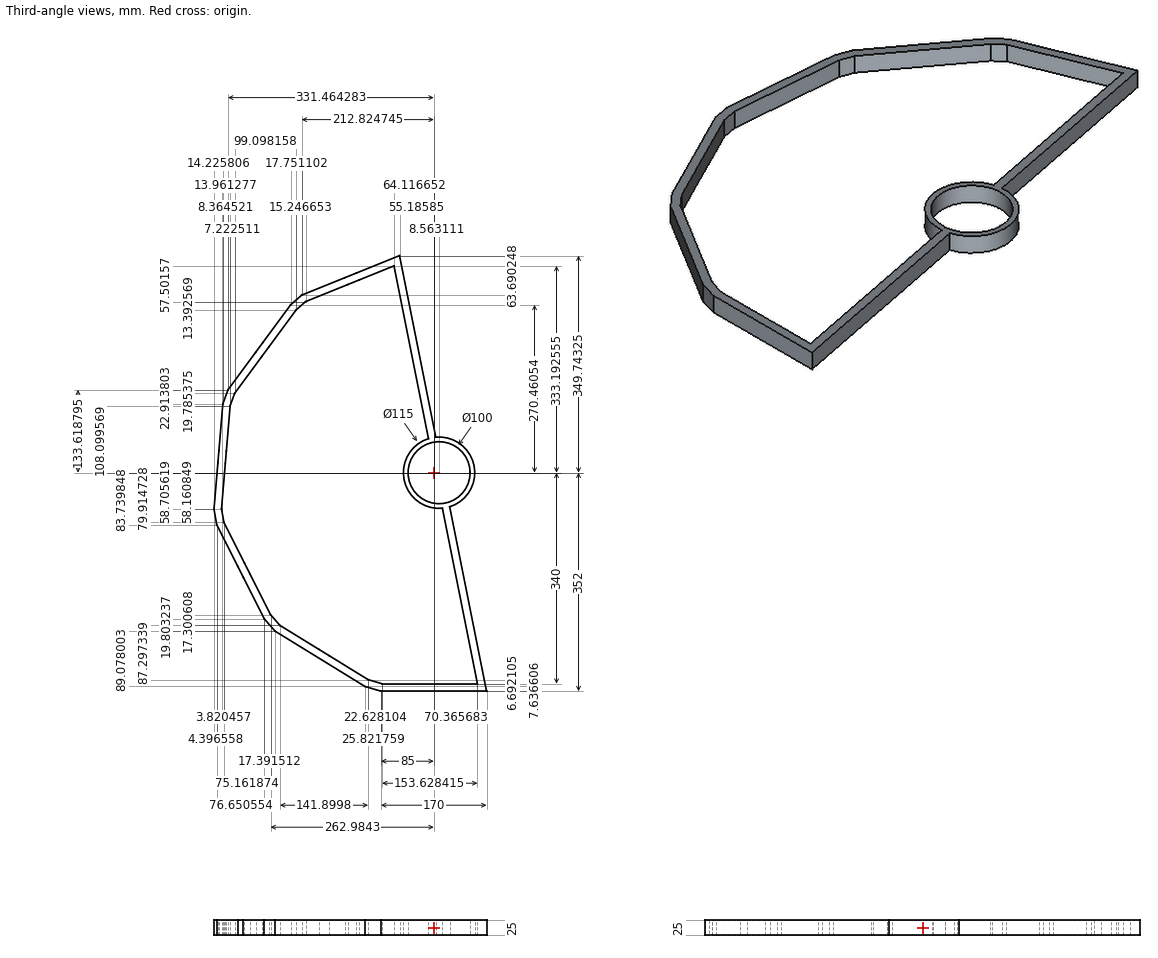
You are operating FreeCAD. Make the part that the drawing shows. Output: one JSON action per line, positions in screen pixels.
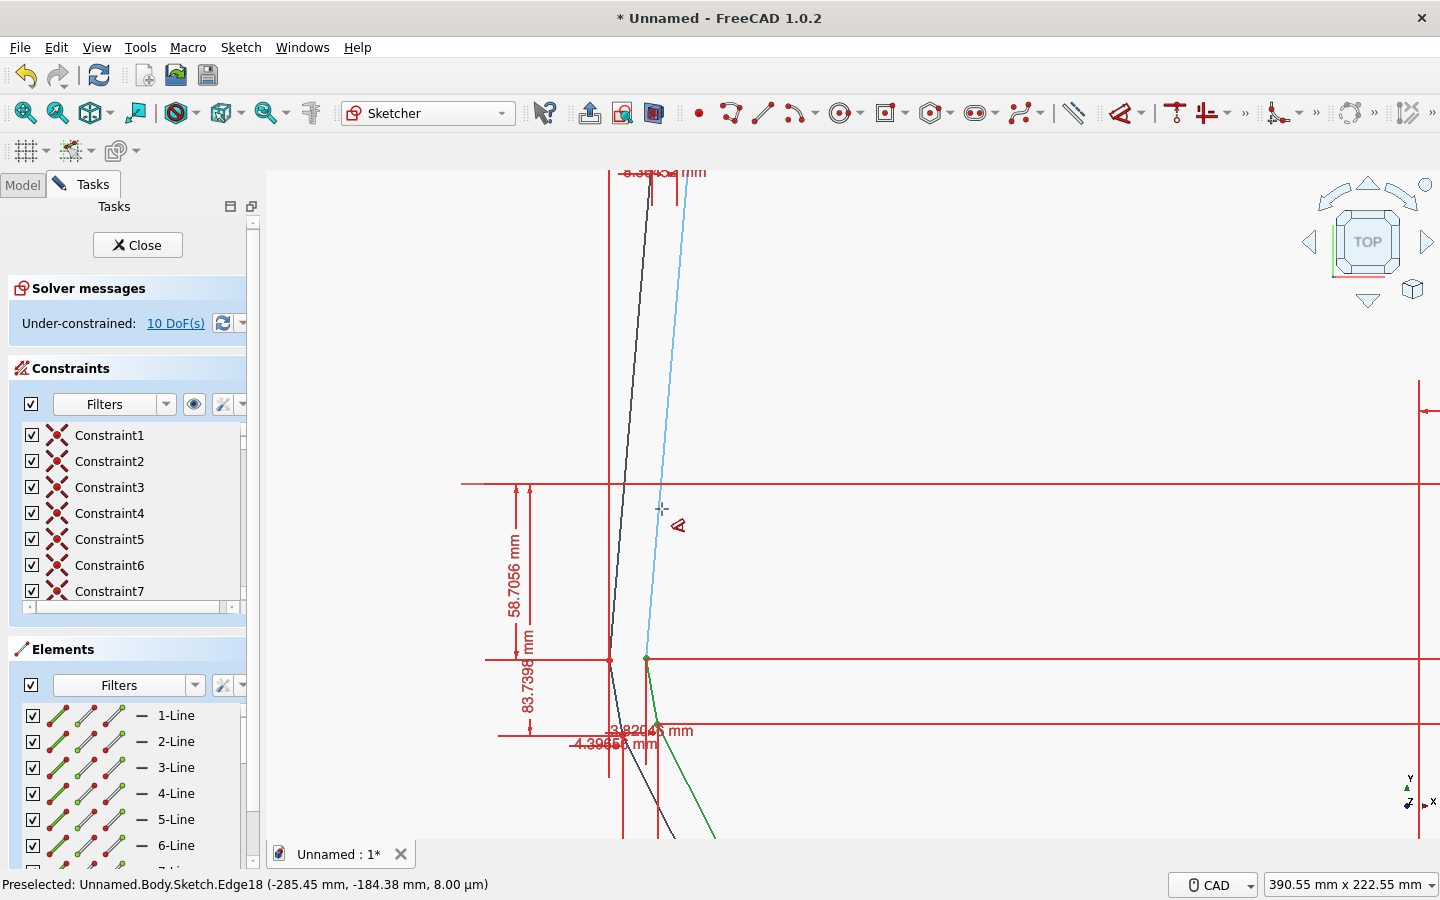
{"action": "left_click", "coordinate": [659, 509]}
{"action": "left_click", "coordinate": [667, 693]}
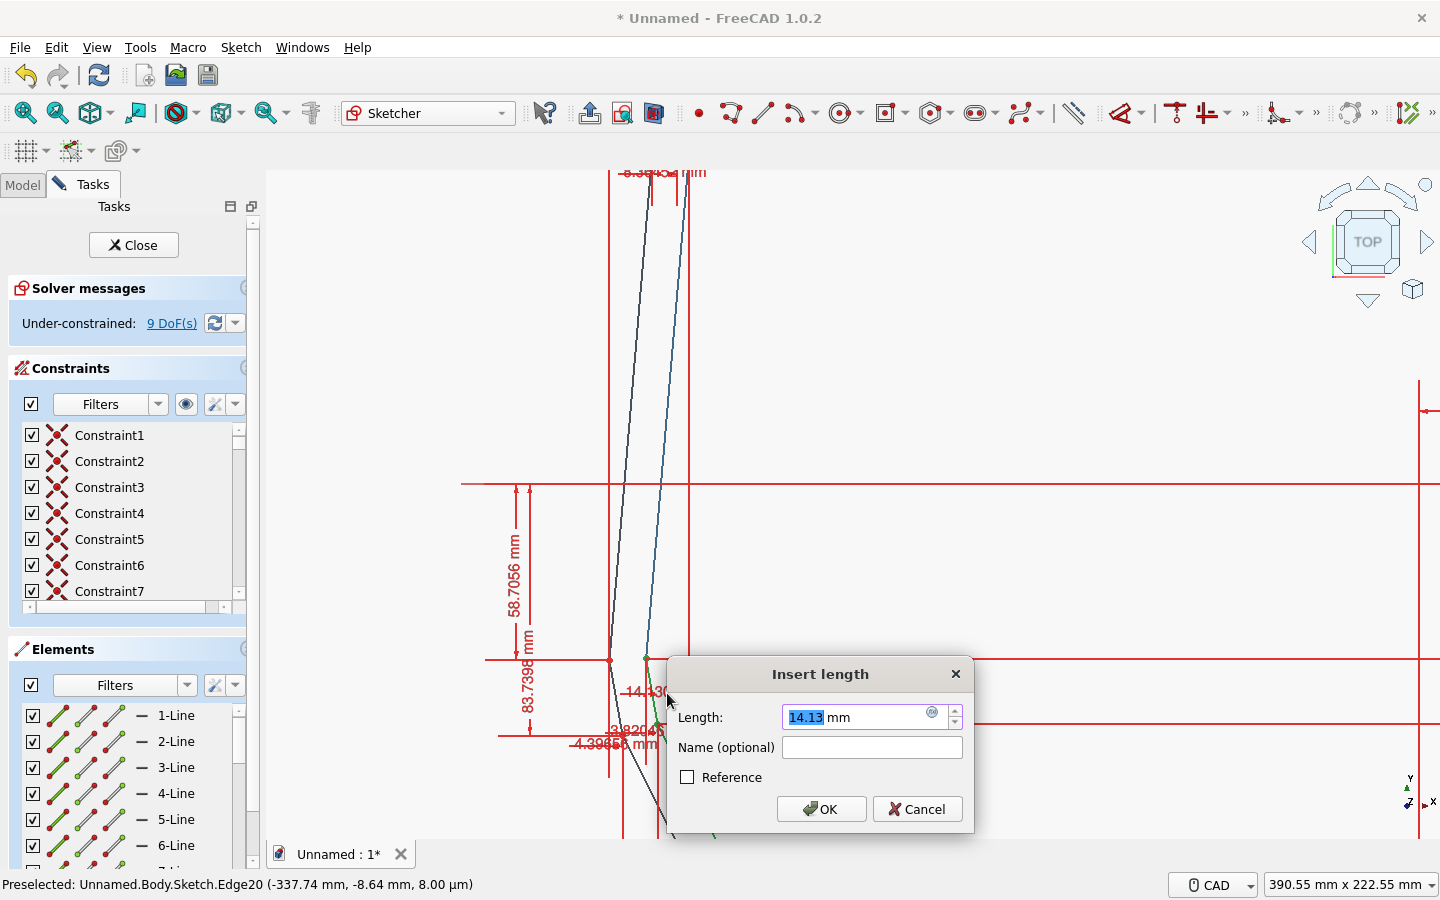
{"action": "type", "text": "13.961277"}
{"action": "key", "text": "Return"}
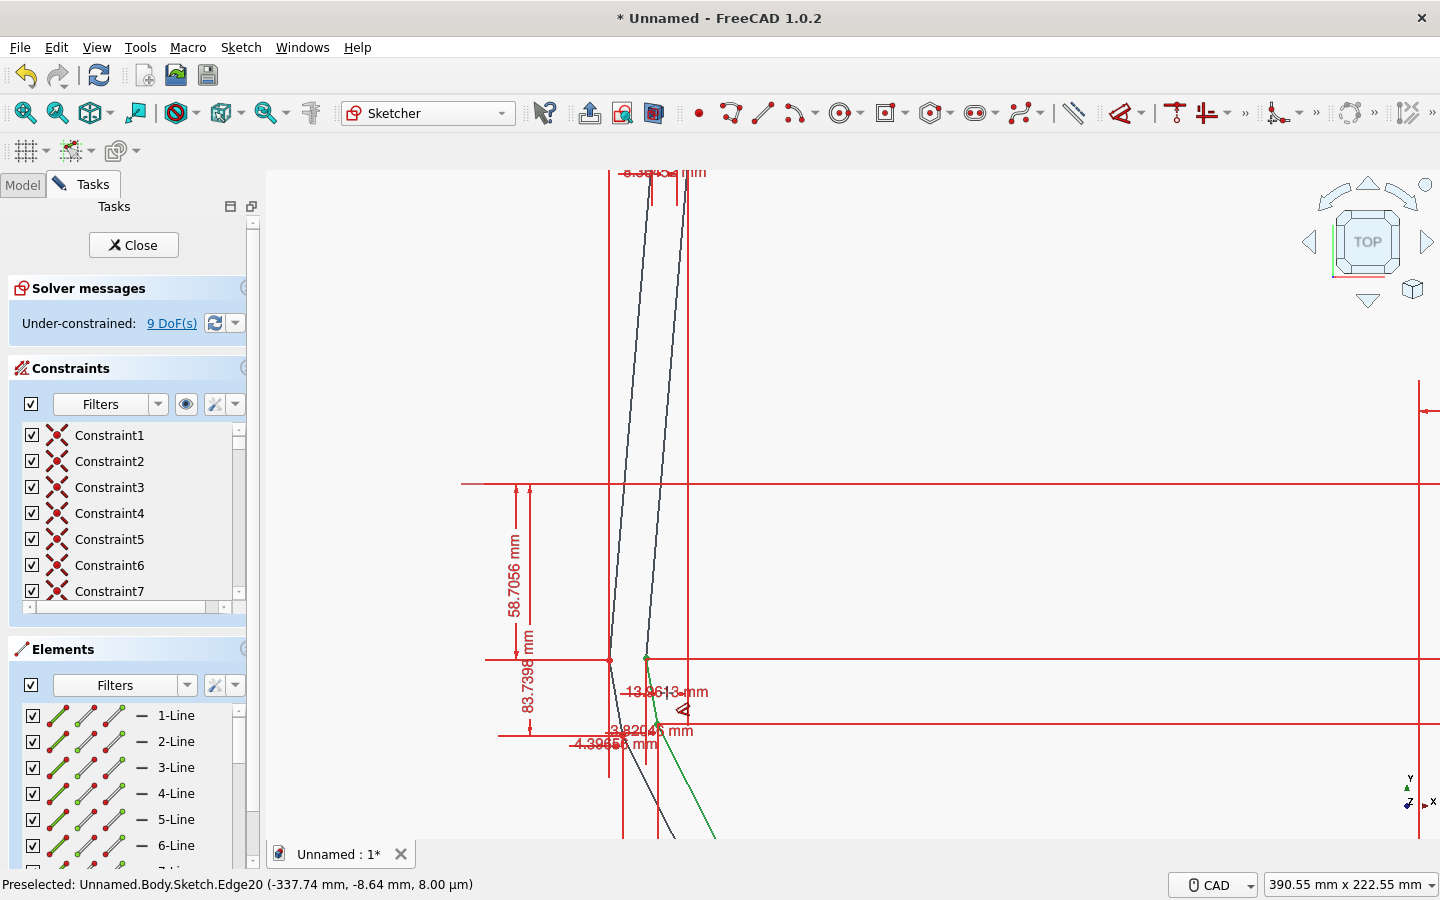
{"action": "scroll", "coordinate": [662, 509], "scroll_direction": "down", "scroll_amount": 8}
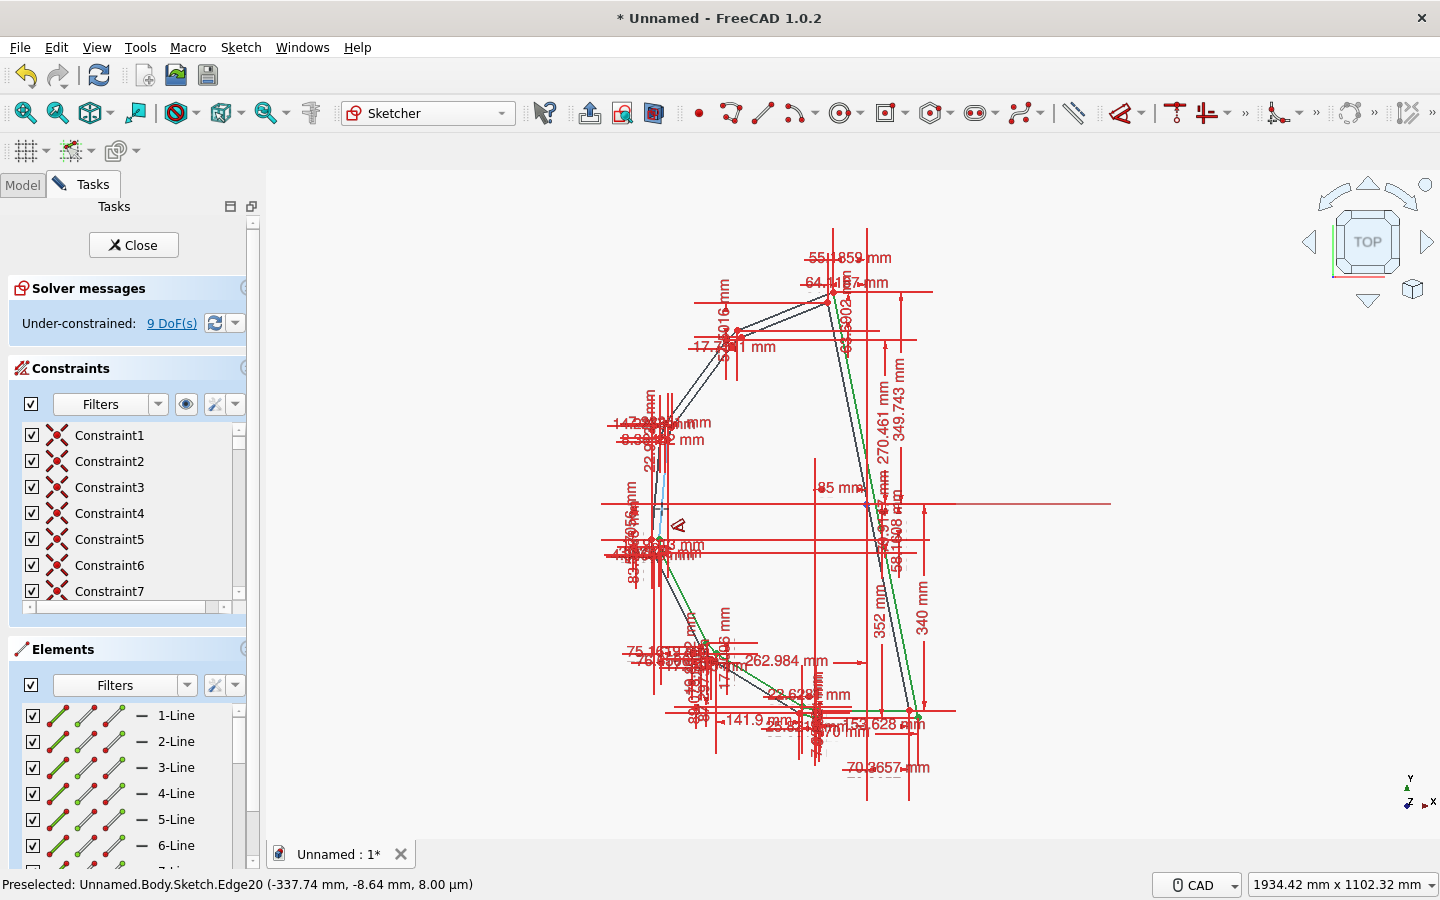
{"action": "scroll", "coordinate": [669, 436], "scroll_direction": "up", "scroll_amount": 7}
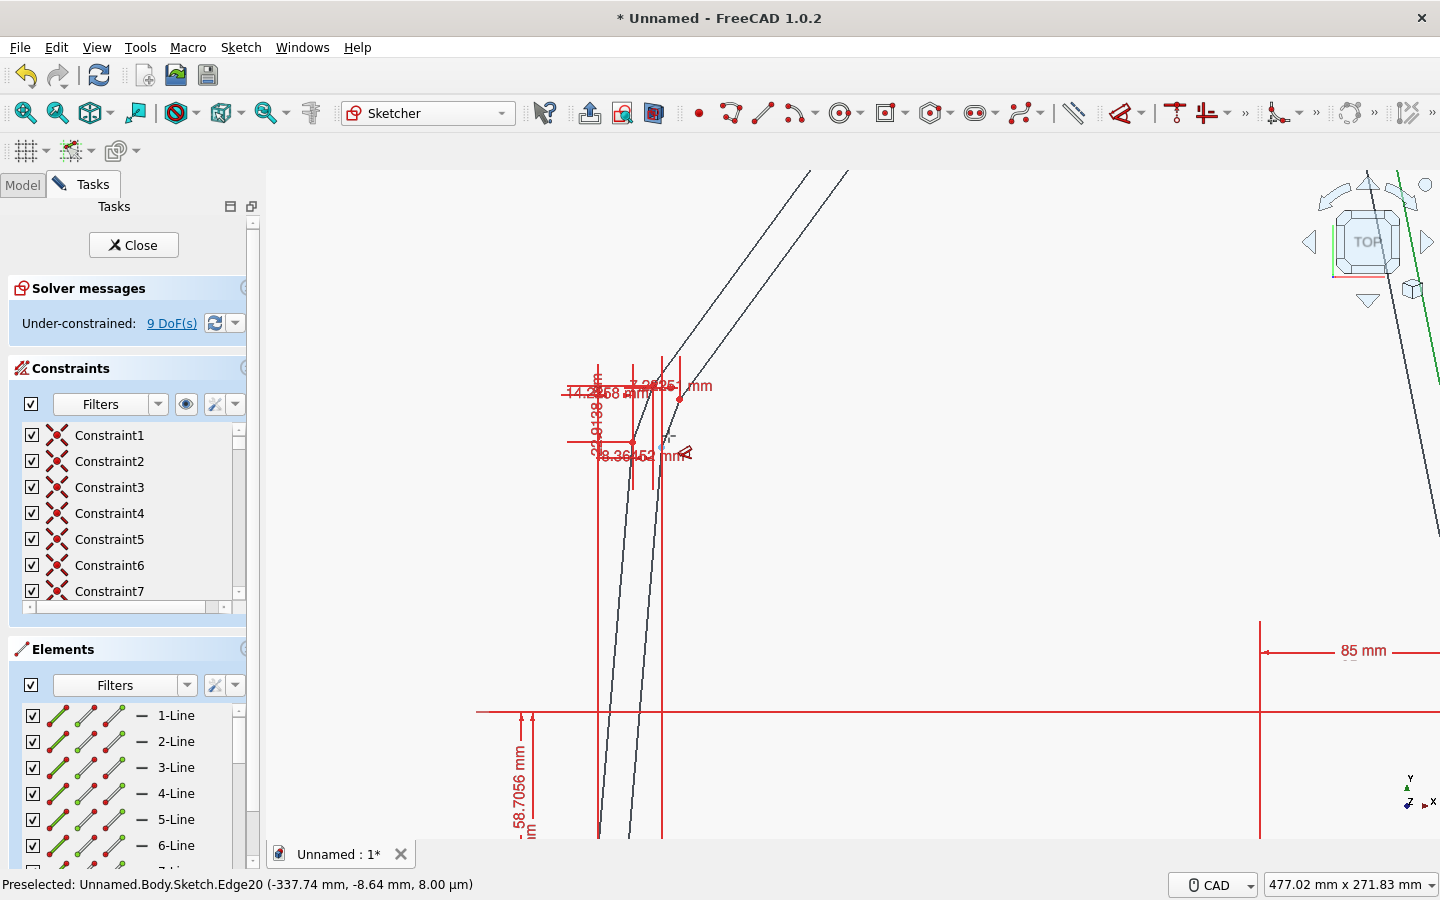
{"action": "left_click", "coordinate": [667, 433]}
{"action": "left_click", "coordinate": [714, 424]}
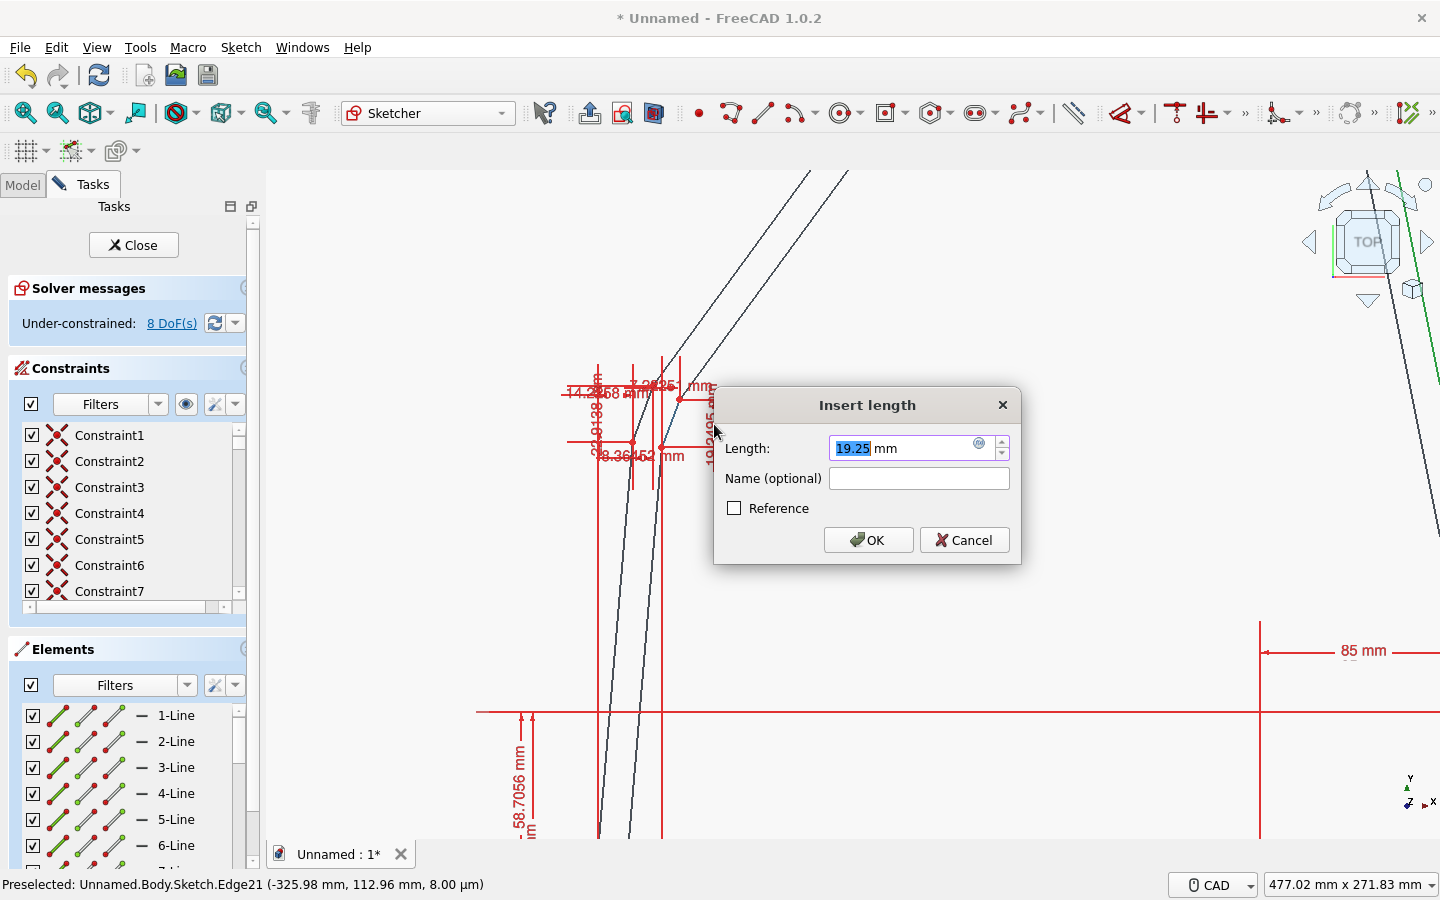
{"action": "type", "text": "19.785375"}
{"action": "key", "text": "Return"}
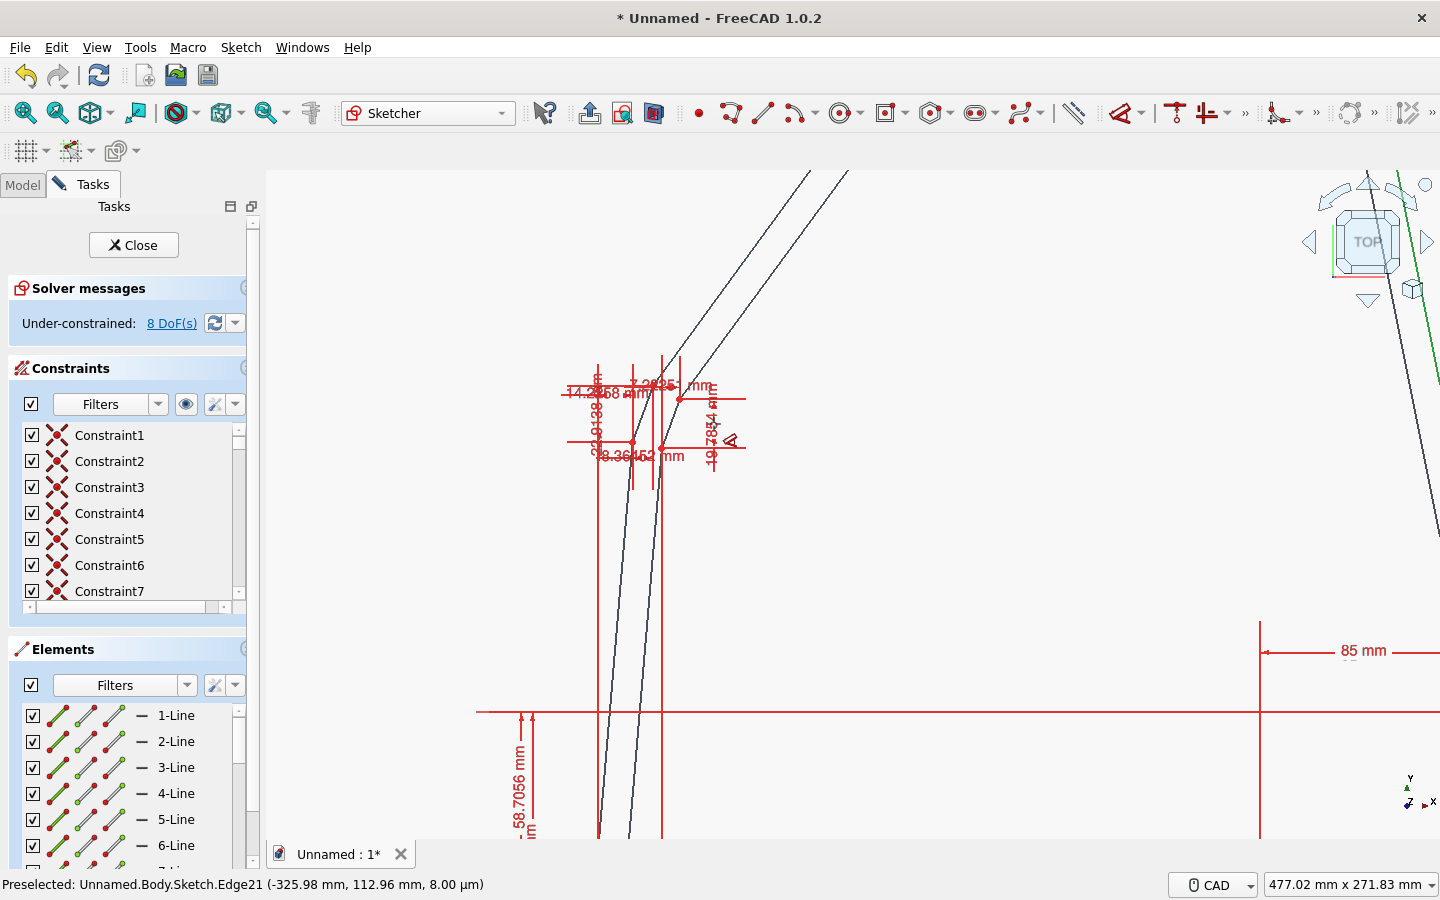
{"action": "left_click", "coordinate": [753, 300]}
{"action": "left_click", "coordinate": [801, 433]}